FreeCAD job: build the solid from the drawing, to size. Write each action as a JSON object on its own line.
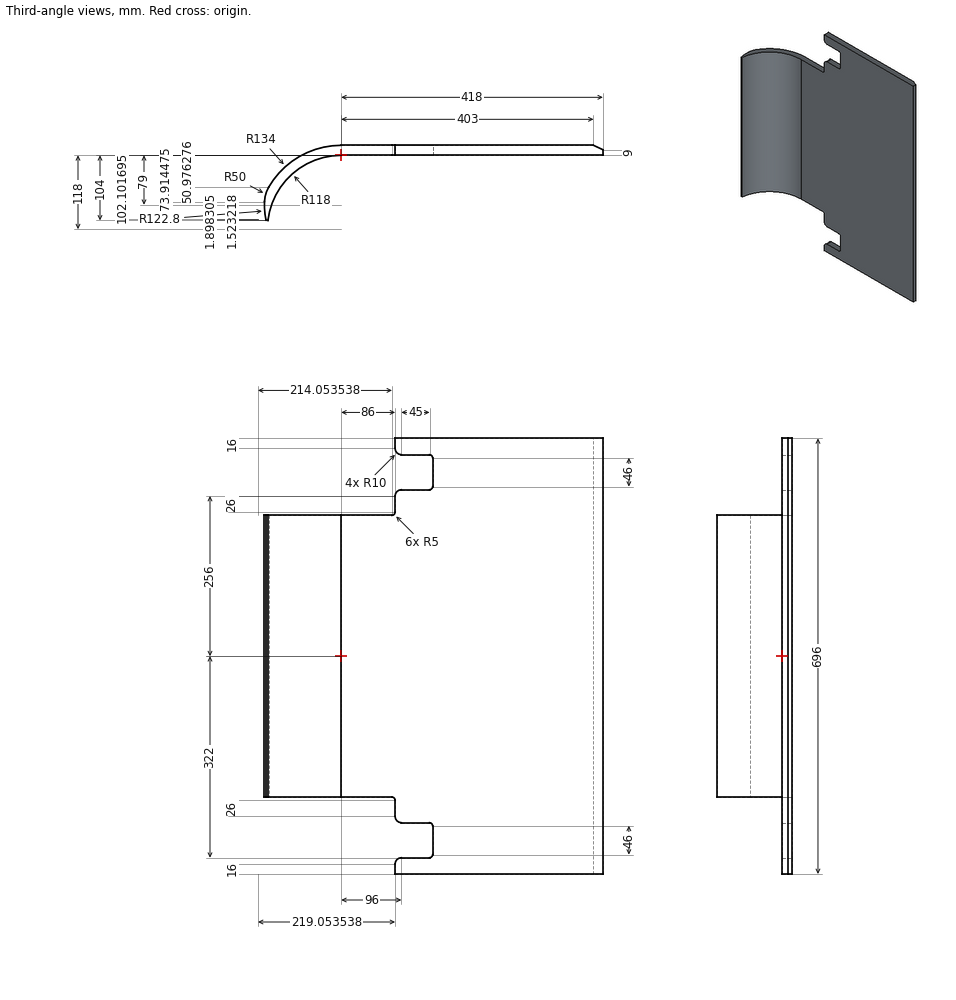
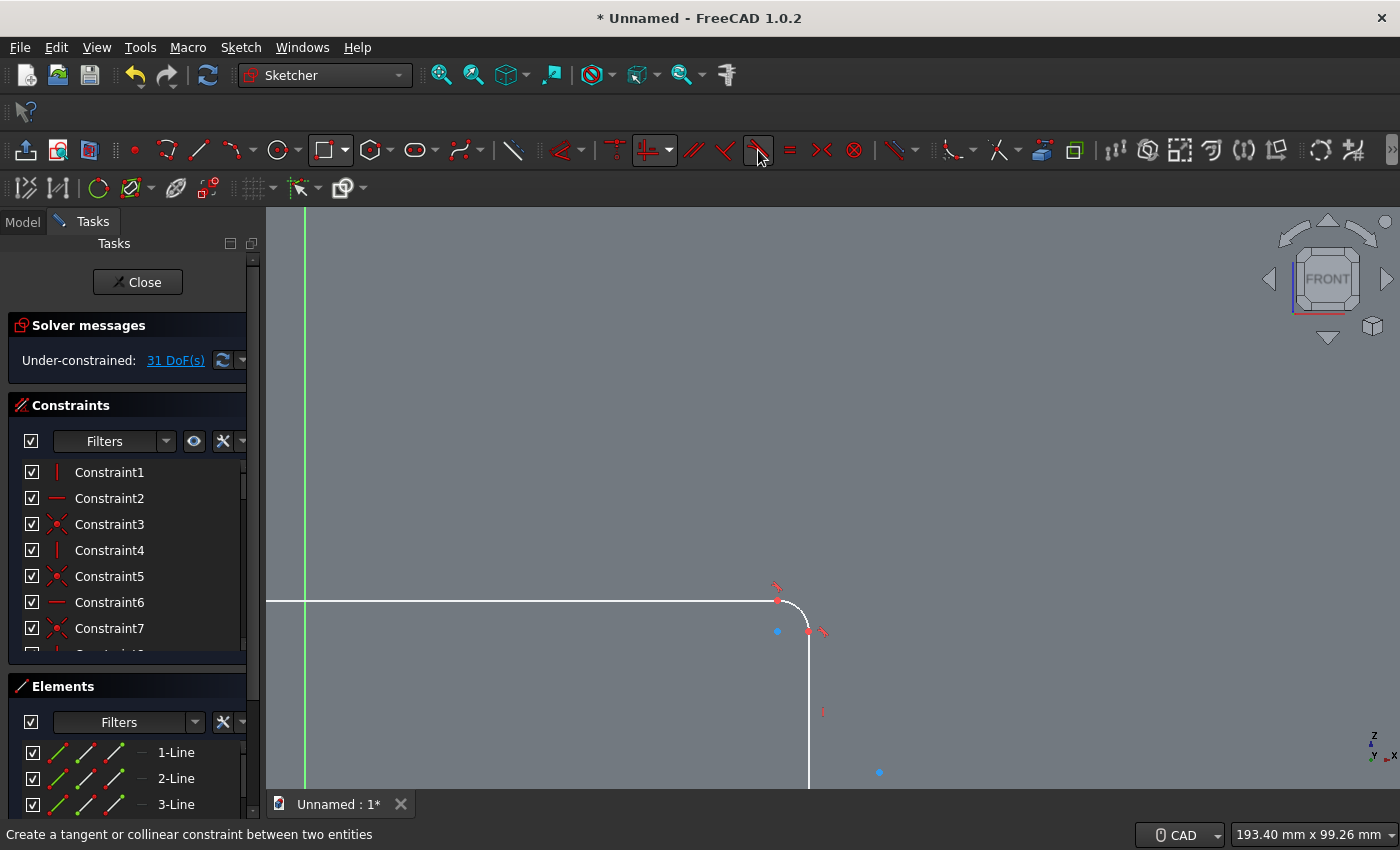
{"action": "scroll", "coordinate": [807, 619], "scroll_direction": "down", "scroll_amount": 12}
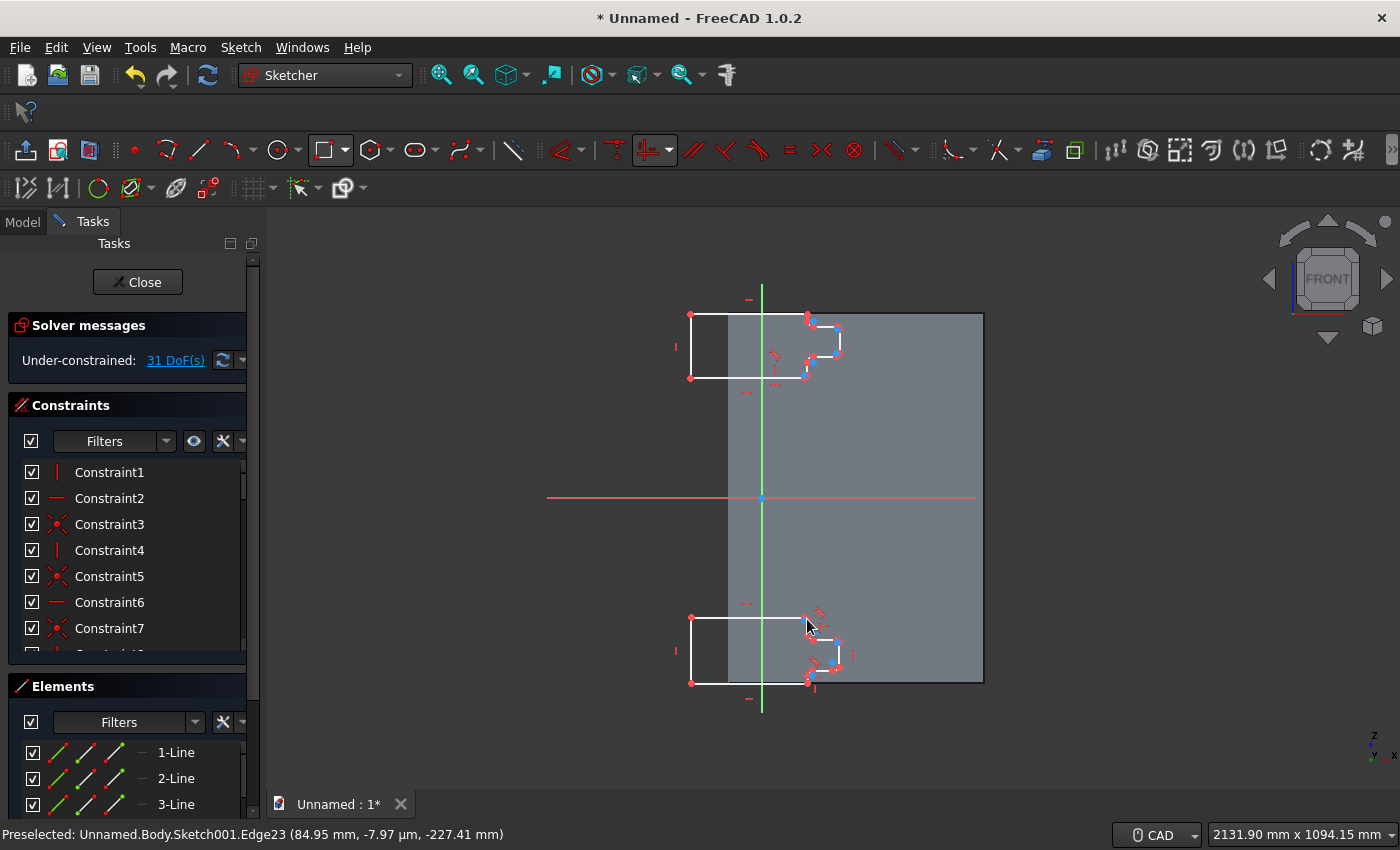
{"action": "scroll", "coordinate": [808, 625], "scroll_direction": "up", "scroll_amount": 6}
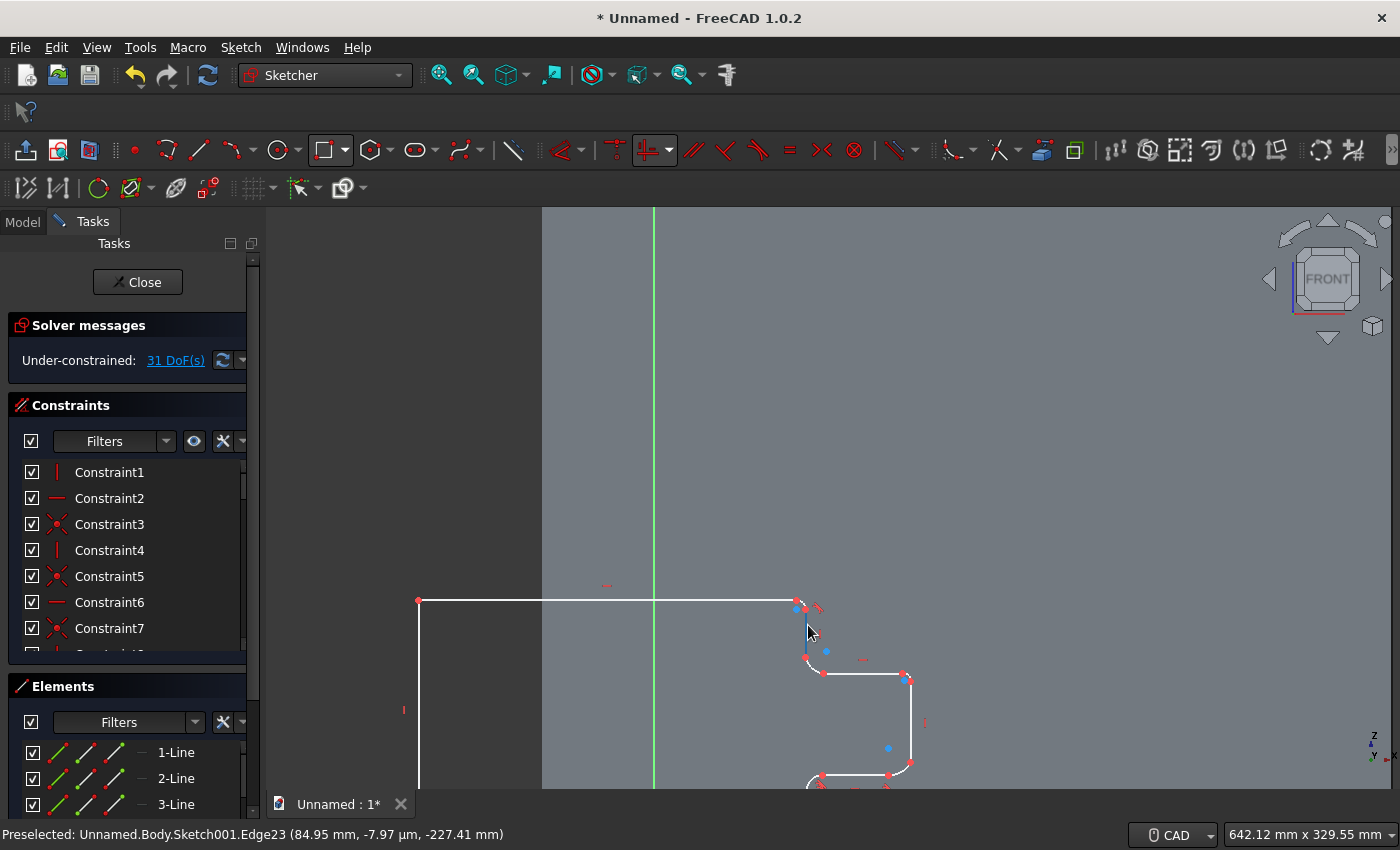
{"action": "left_click", "coordinate": [806, 624]}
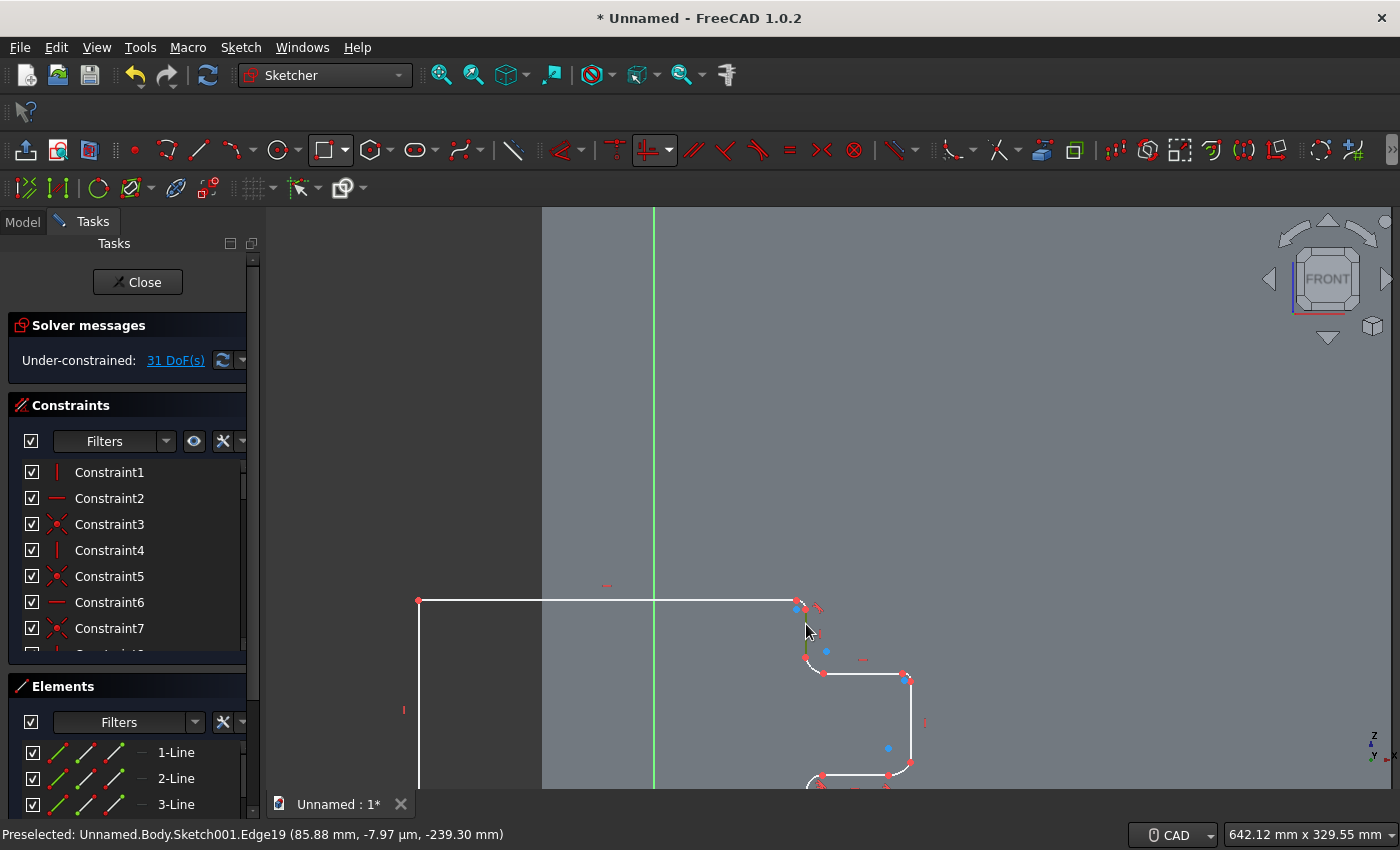
{"action": "left_click", "coordinate": [812, 668]}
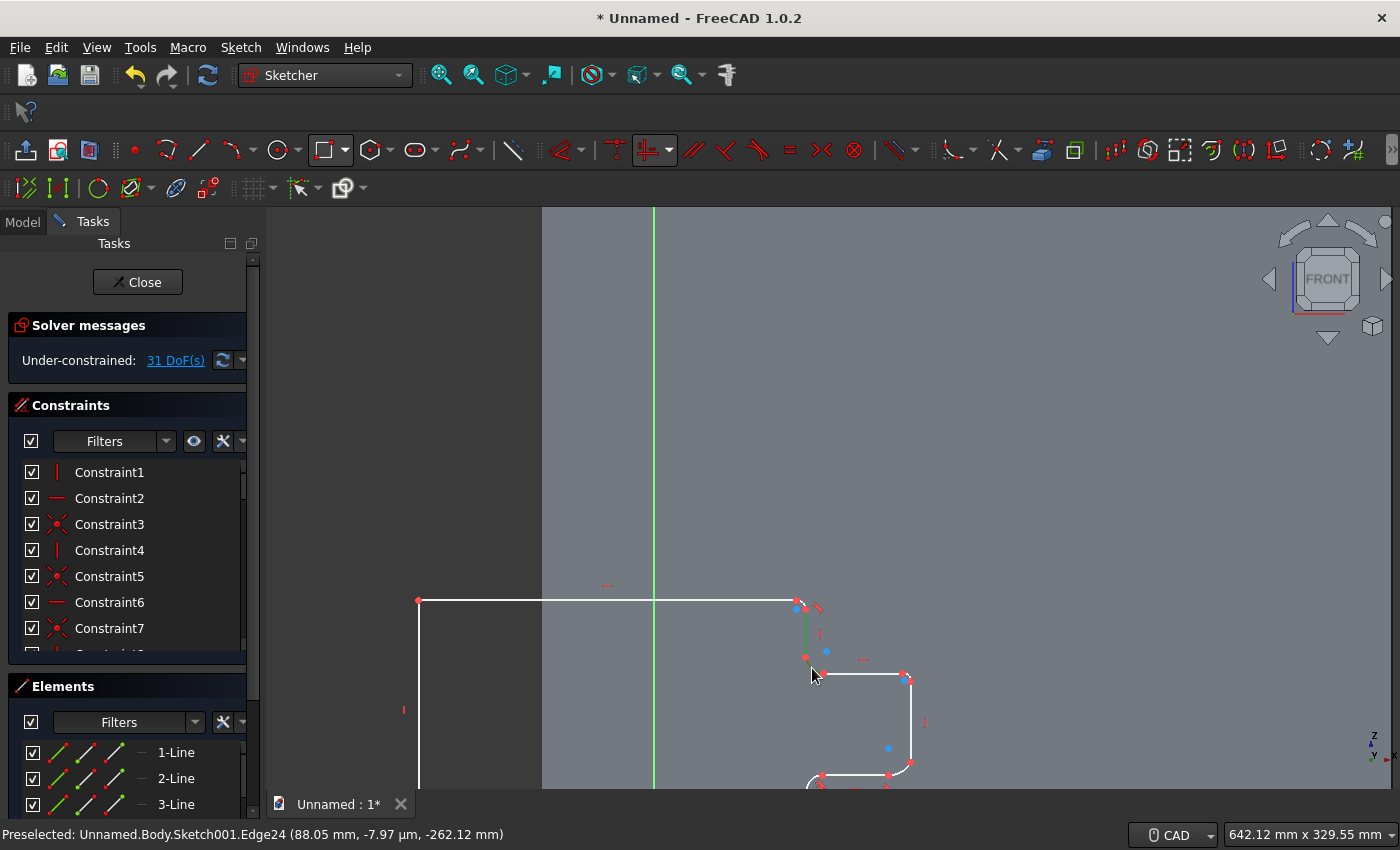
{"action": "left_click", "coordinate": [758, 150]}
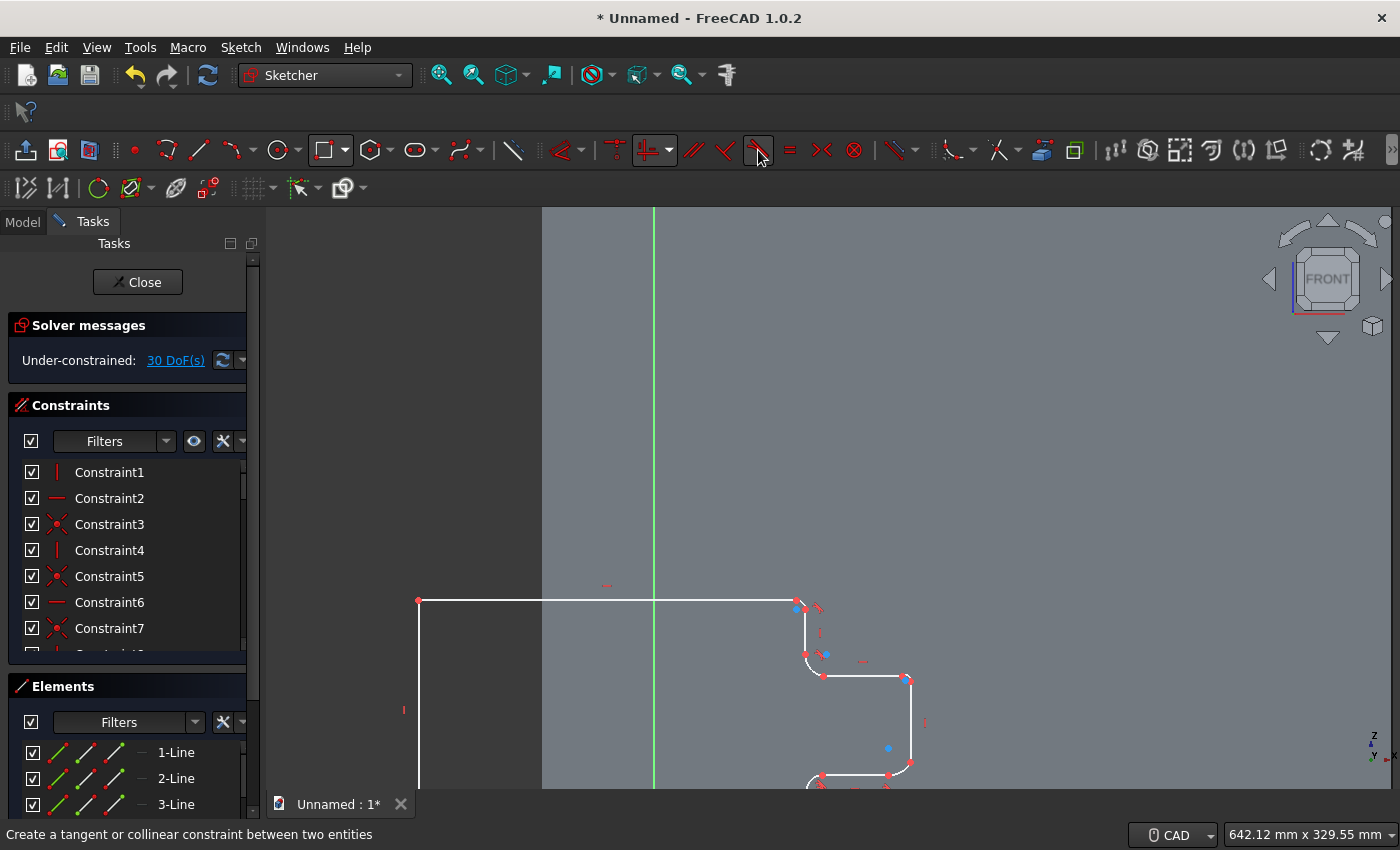
{"action": "left_click", "coordinate": [847, 676]}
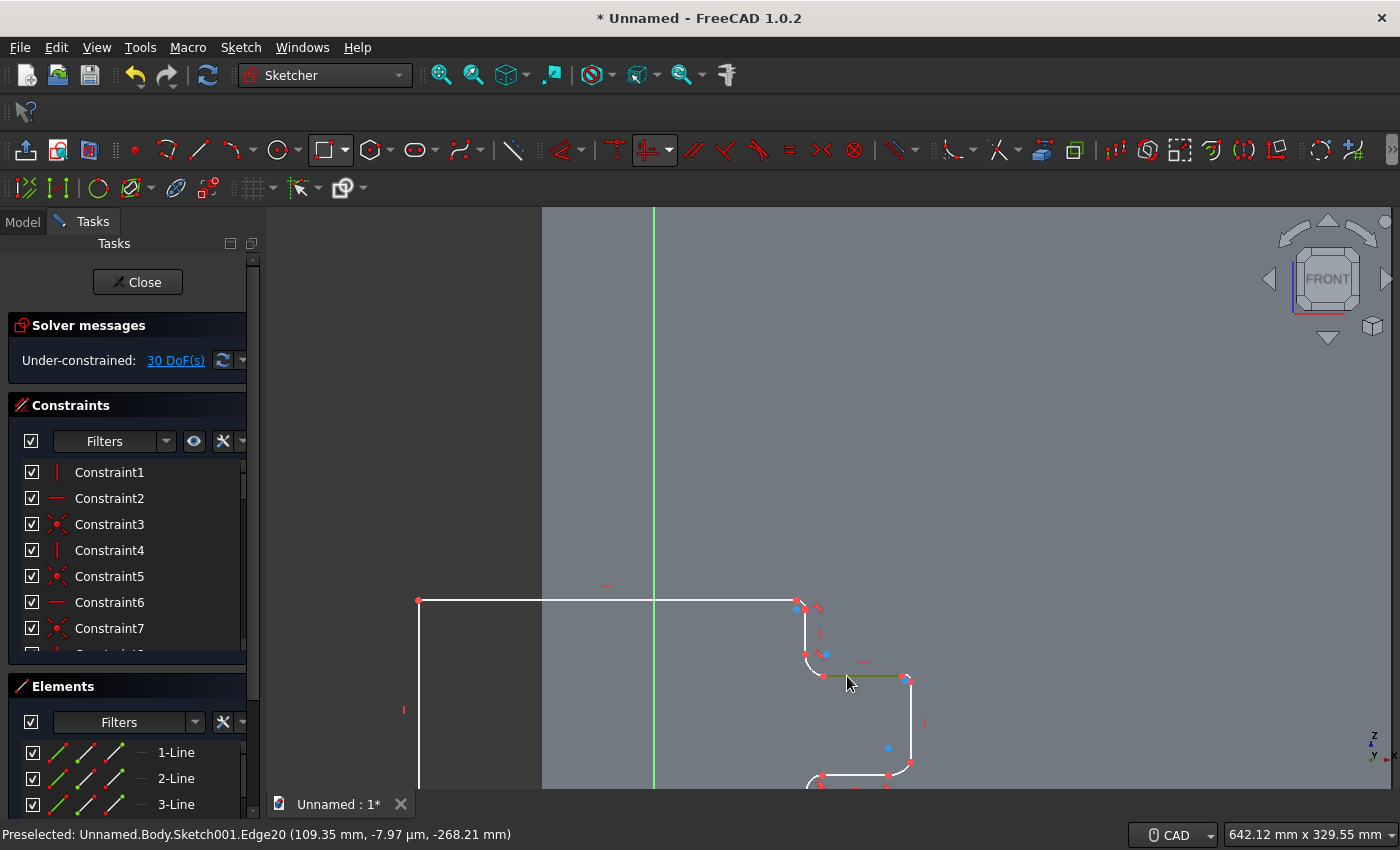
{"action": "scroll", "coordinate": [807, 664], "scroll_direction": "up", "scroll_amount": 3}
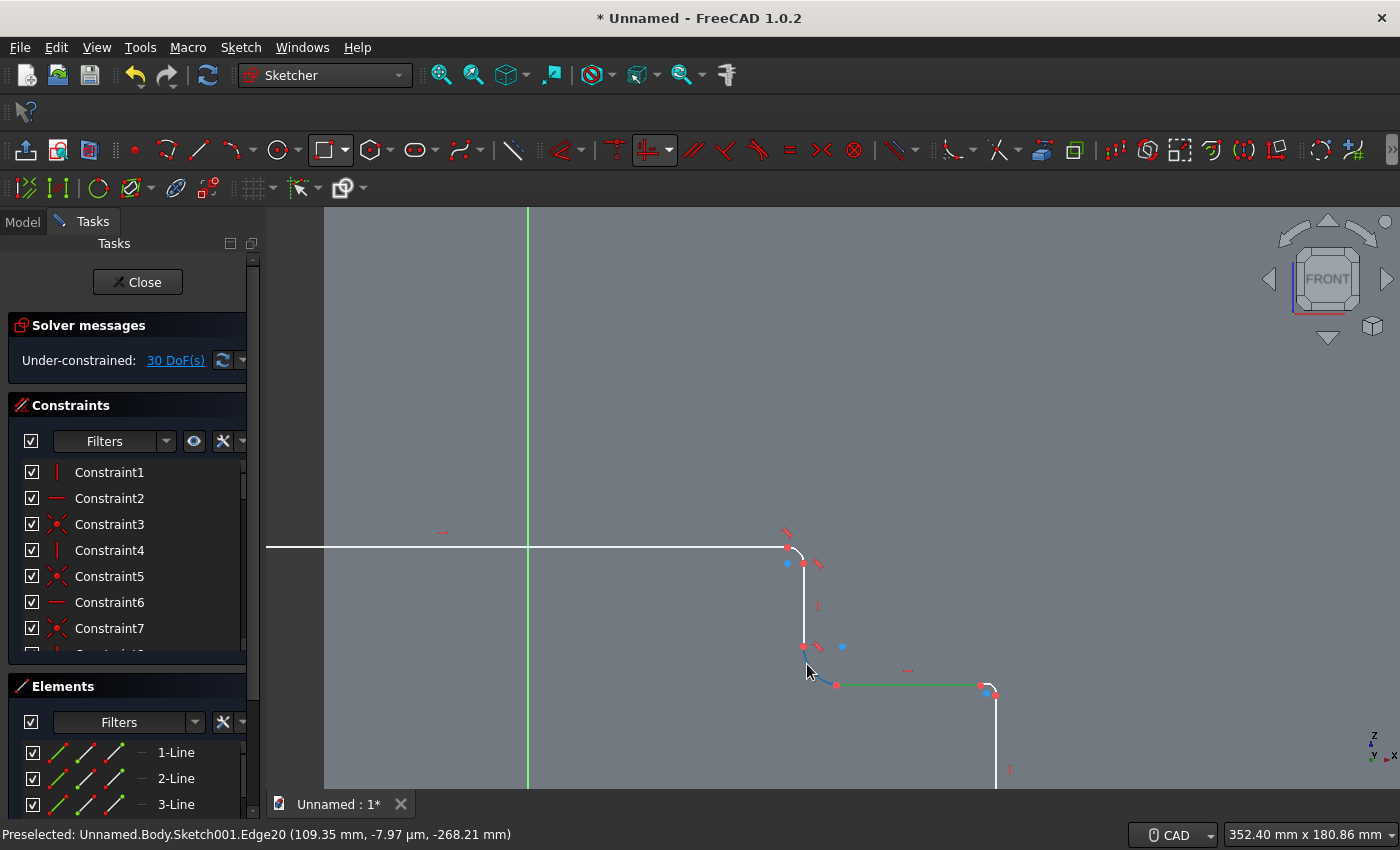
{"action": "left_click", "coordinate": [807, 663]}